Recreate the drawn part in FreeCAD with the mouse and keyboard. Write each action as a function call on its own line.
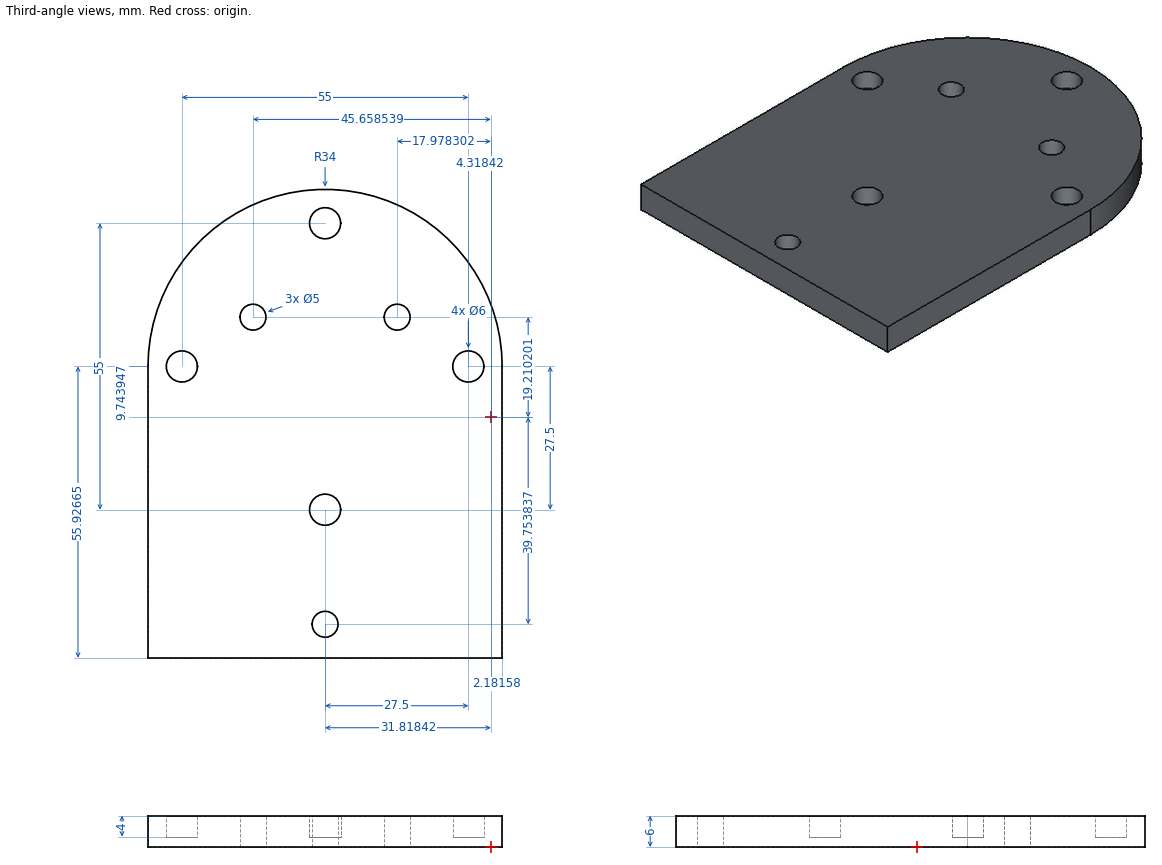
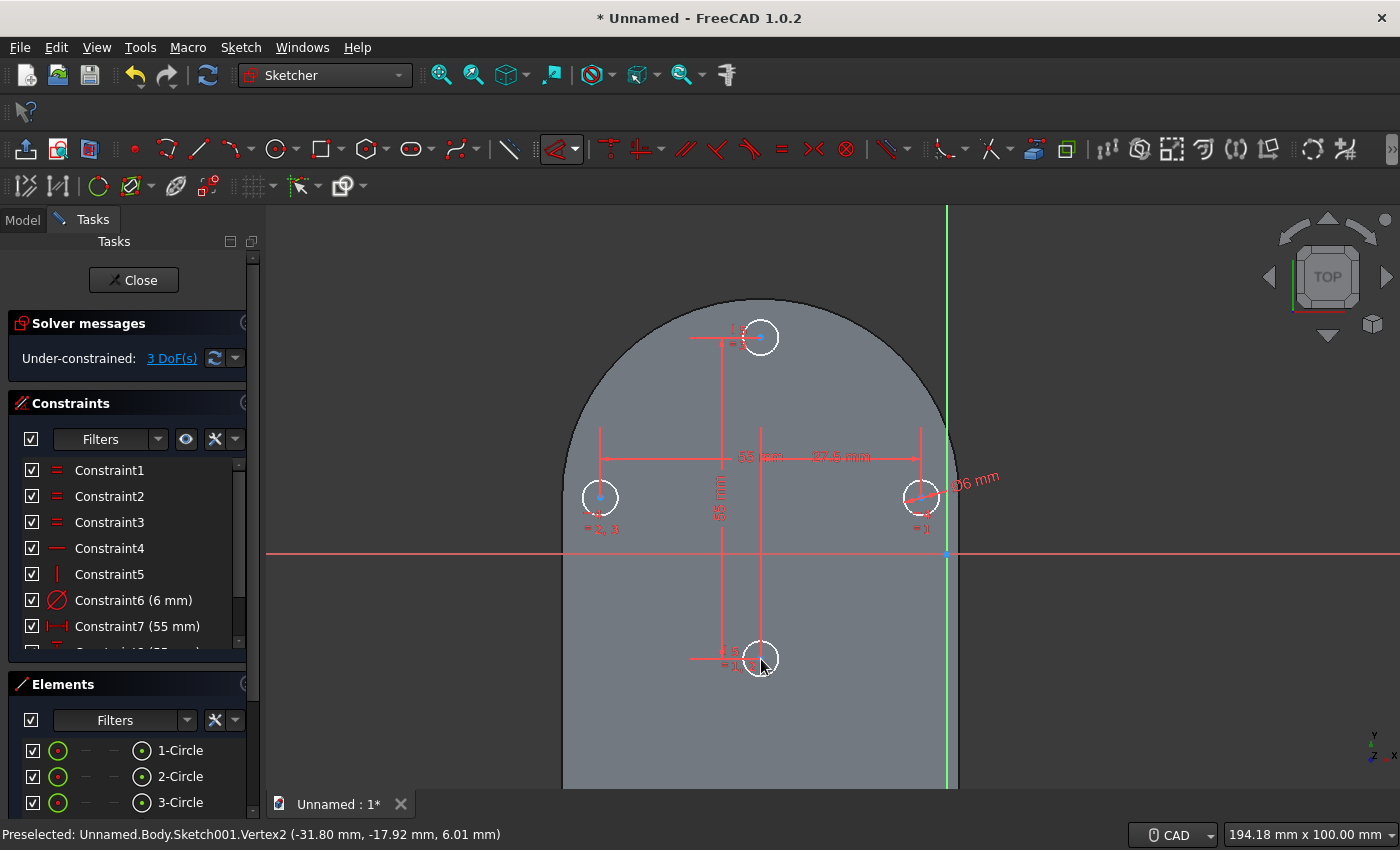
click(921, 498)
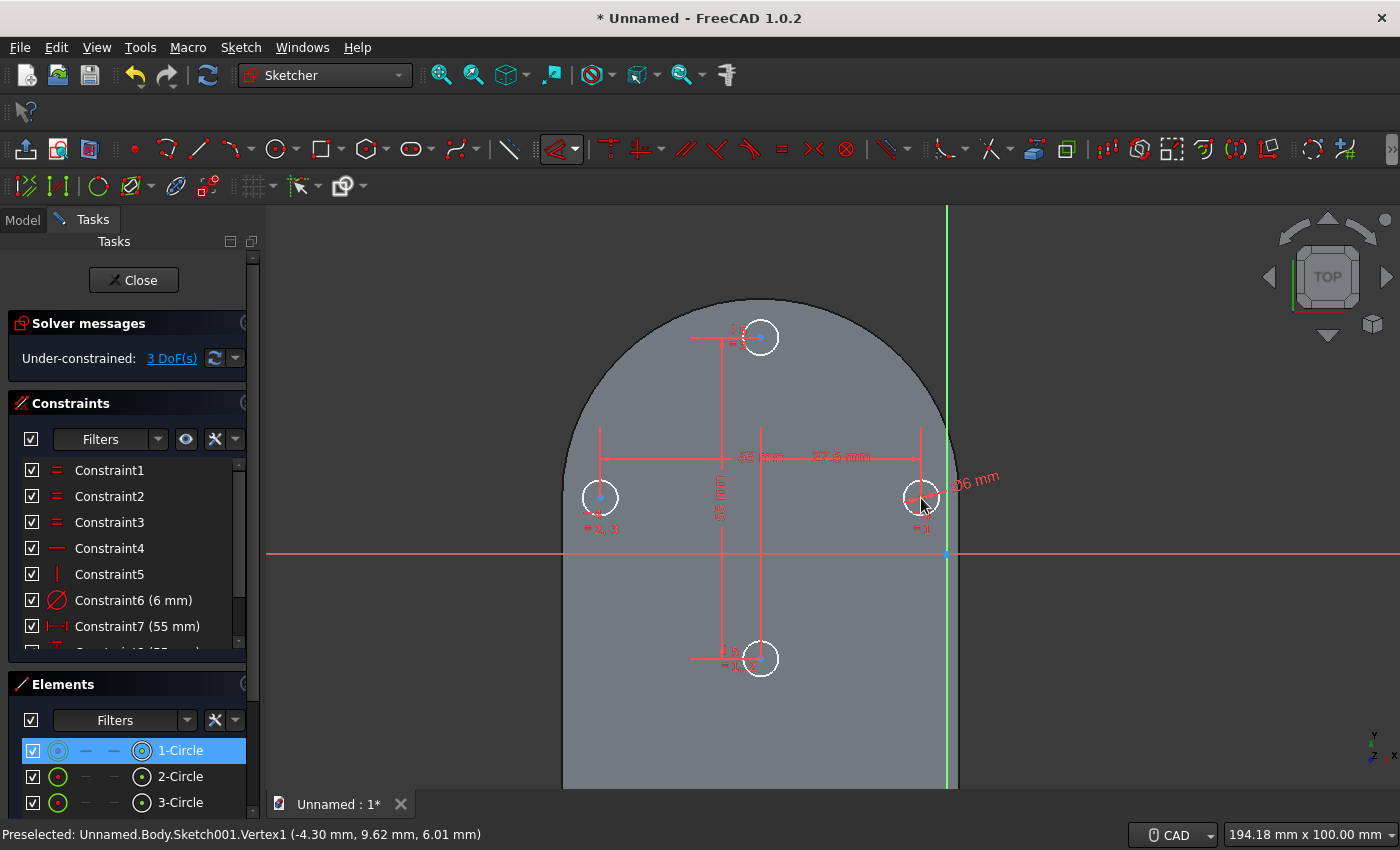
click(761, 659)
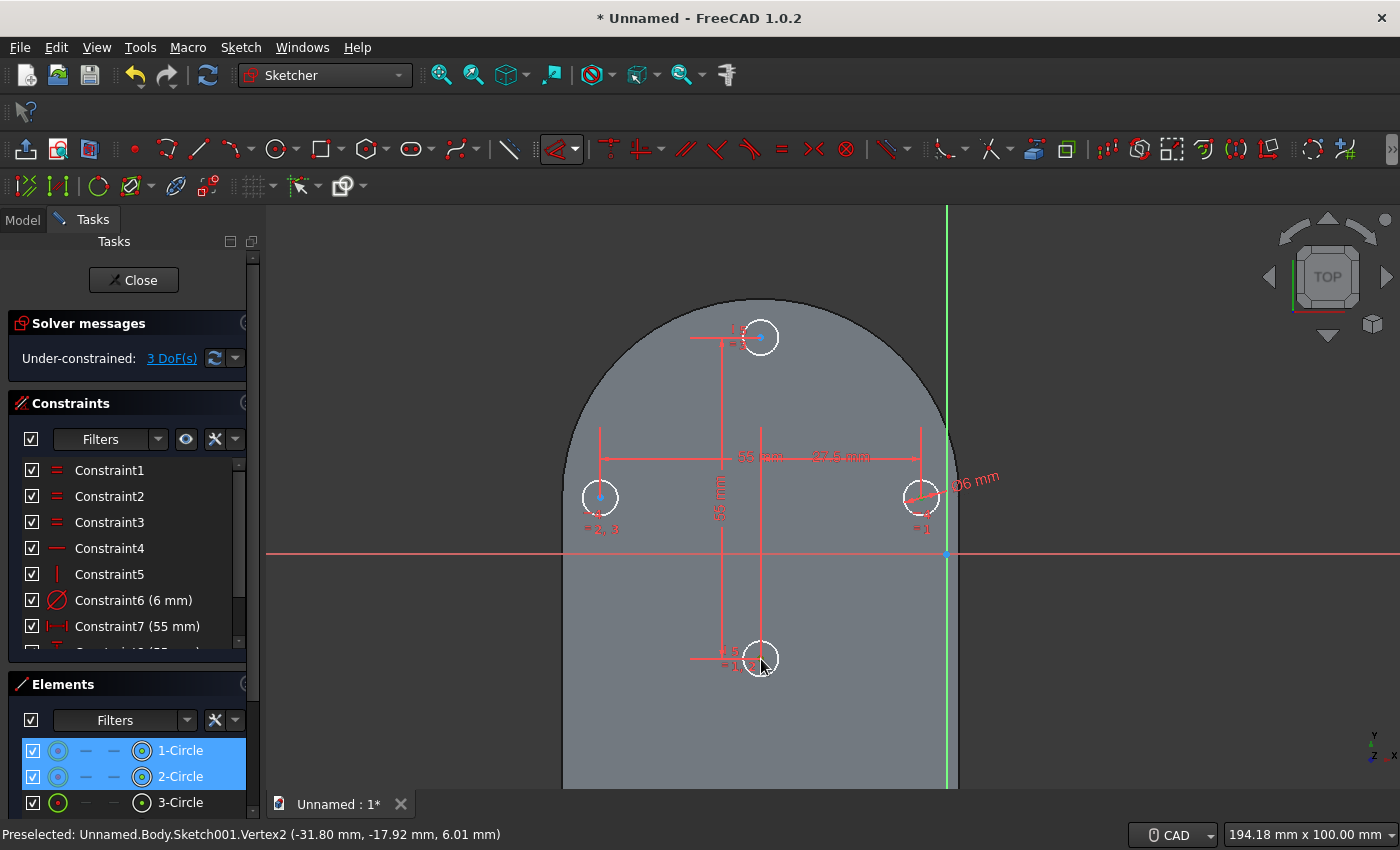
key(i)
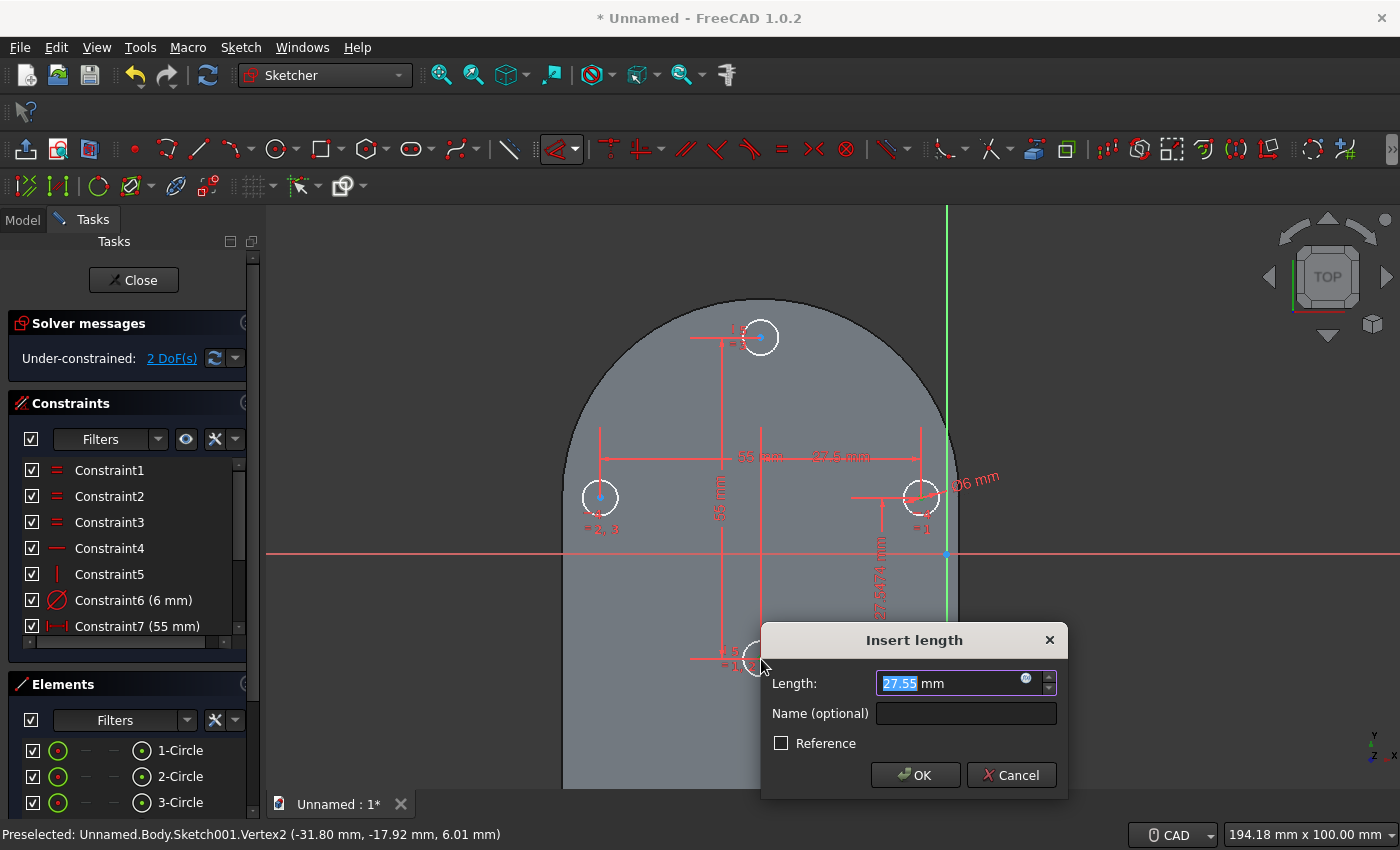
text(27.5)
key(Return)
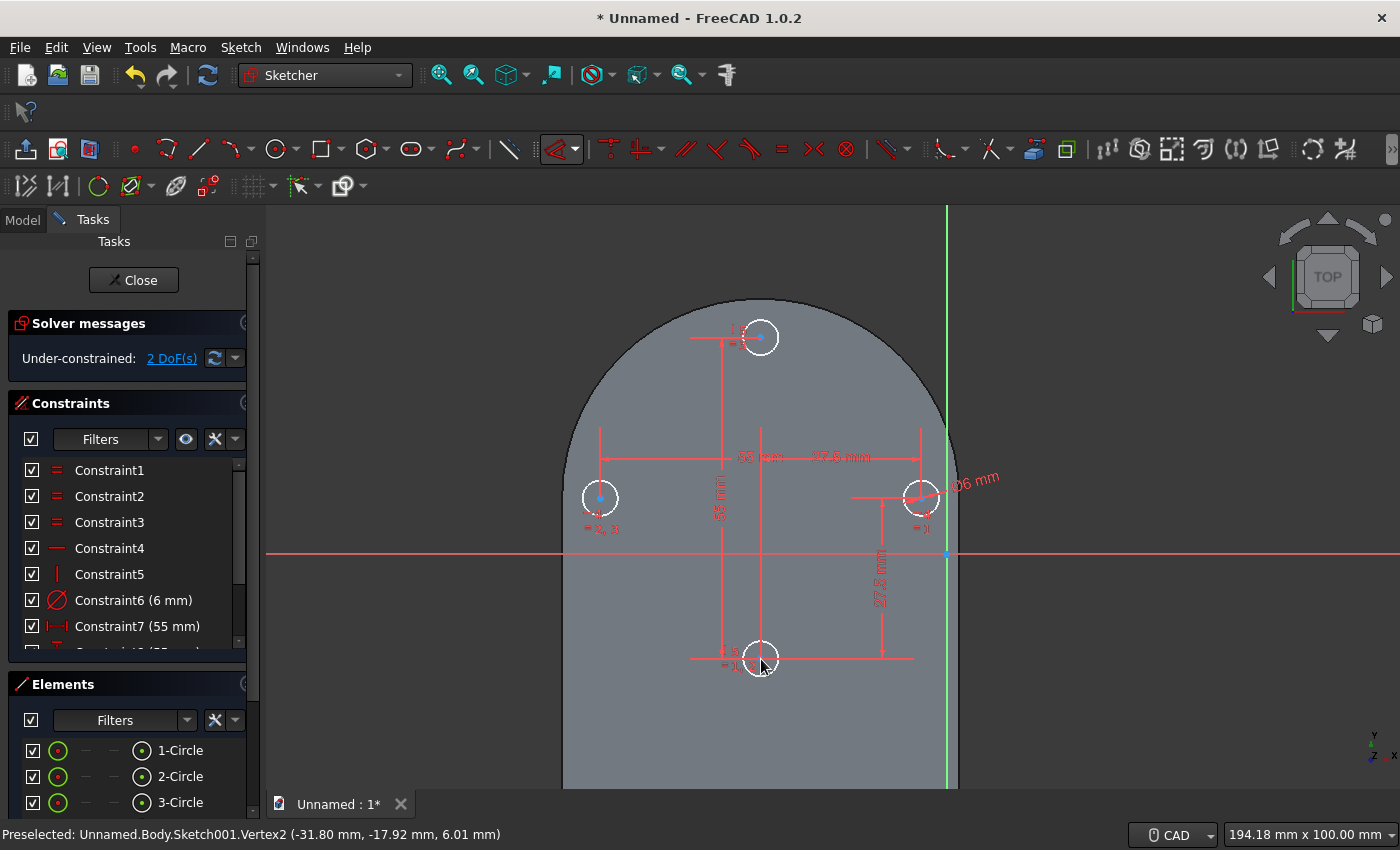
scroll(921, 498, up, 3)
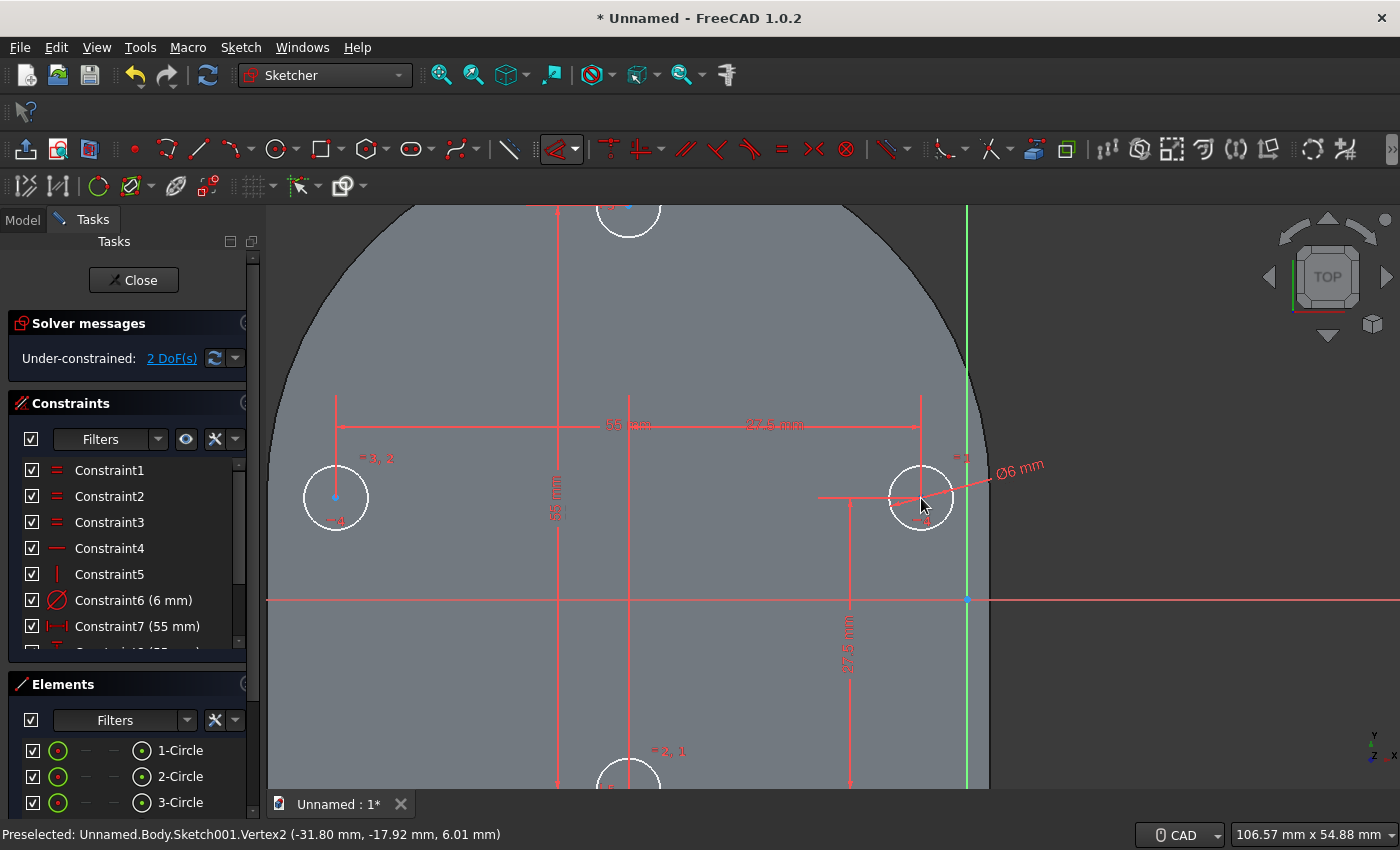
click(921, 498)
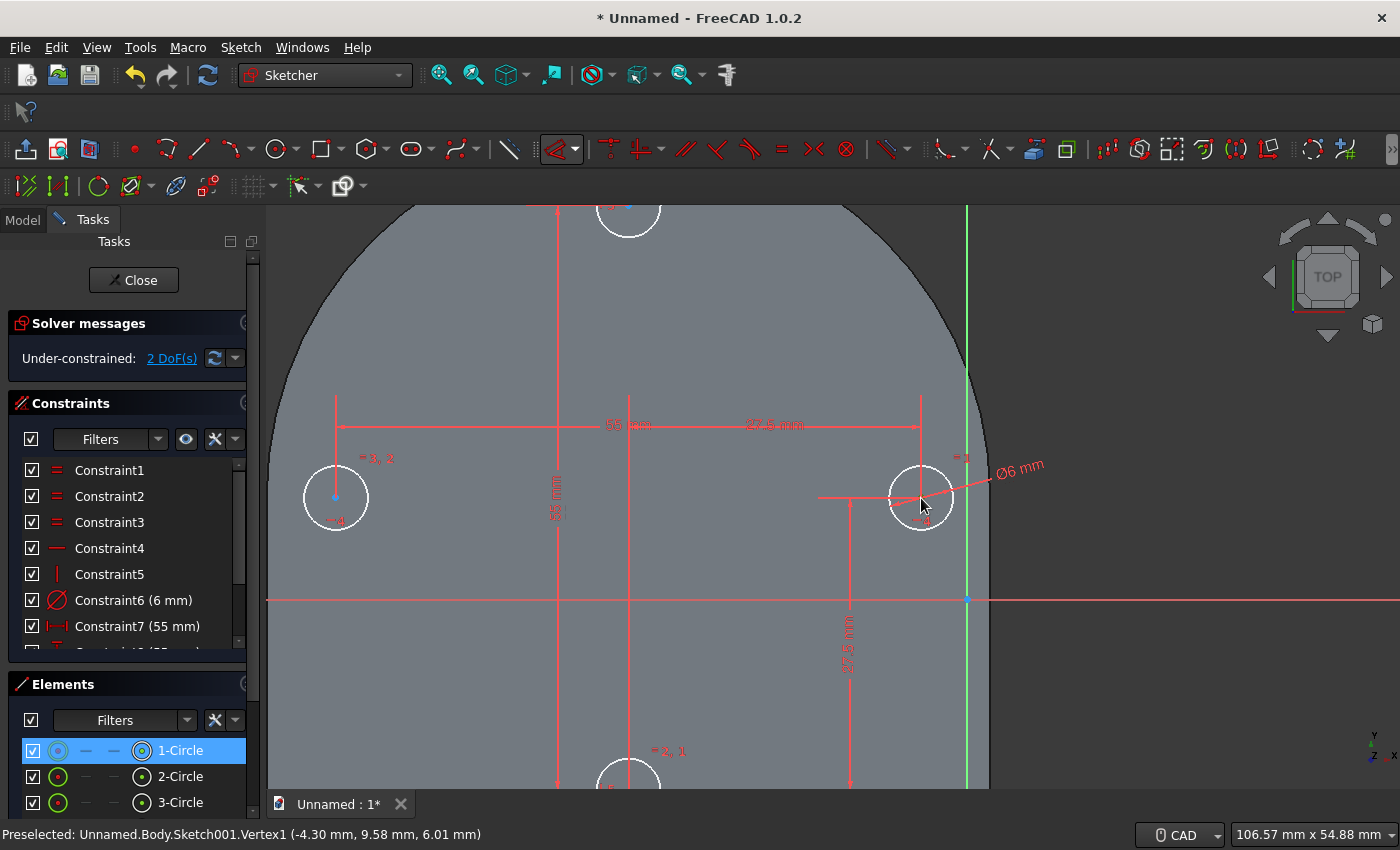
key(l)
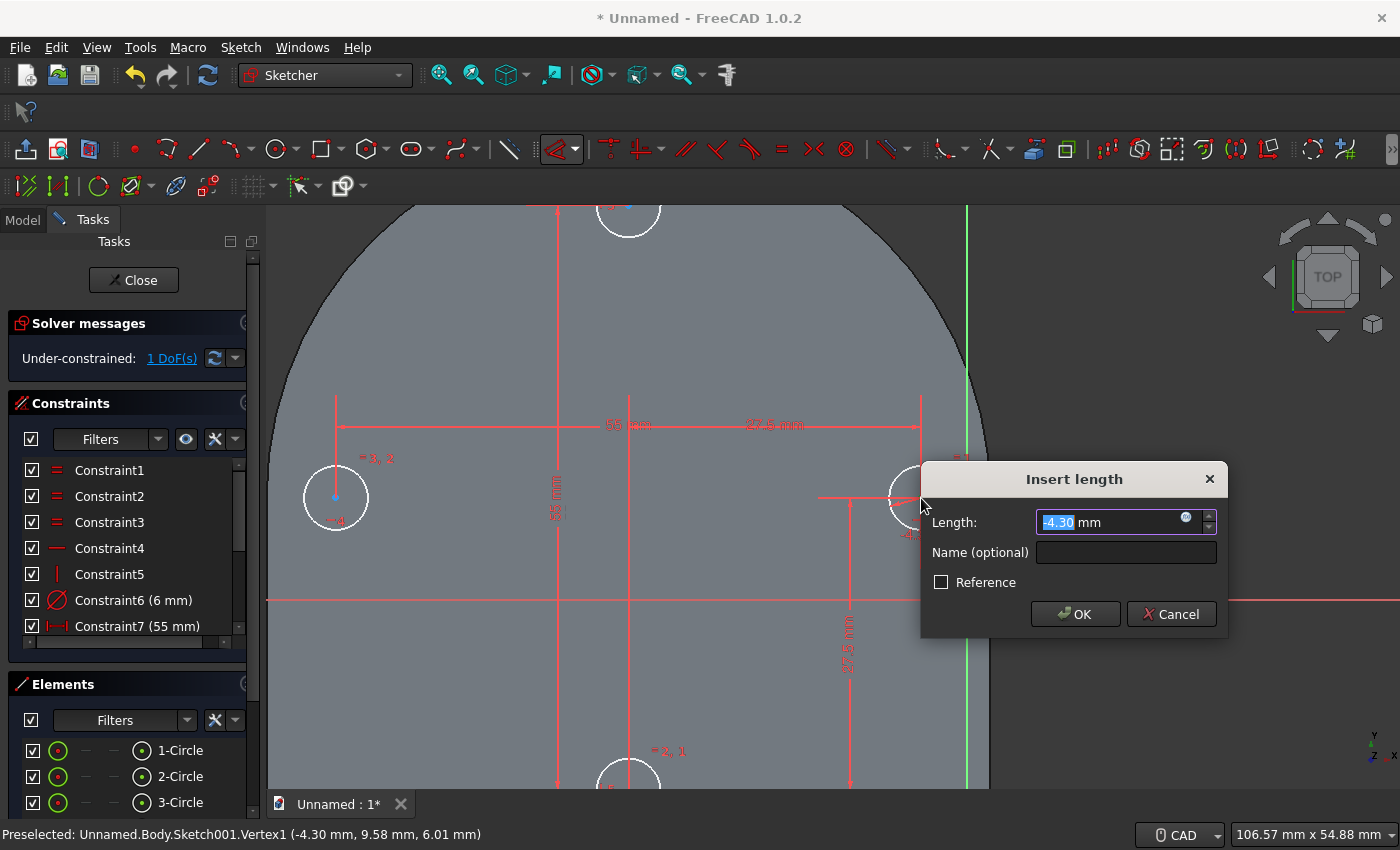
text(-4.31842)
key(Return)